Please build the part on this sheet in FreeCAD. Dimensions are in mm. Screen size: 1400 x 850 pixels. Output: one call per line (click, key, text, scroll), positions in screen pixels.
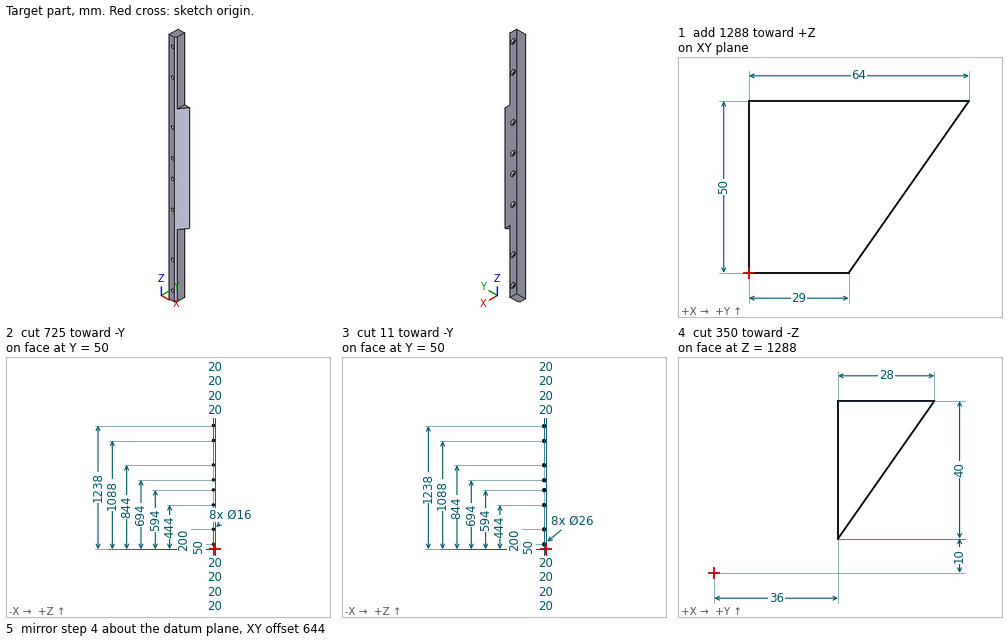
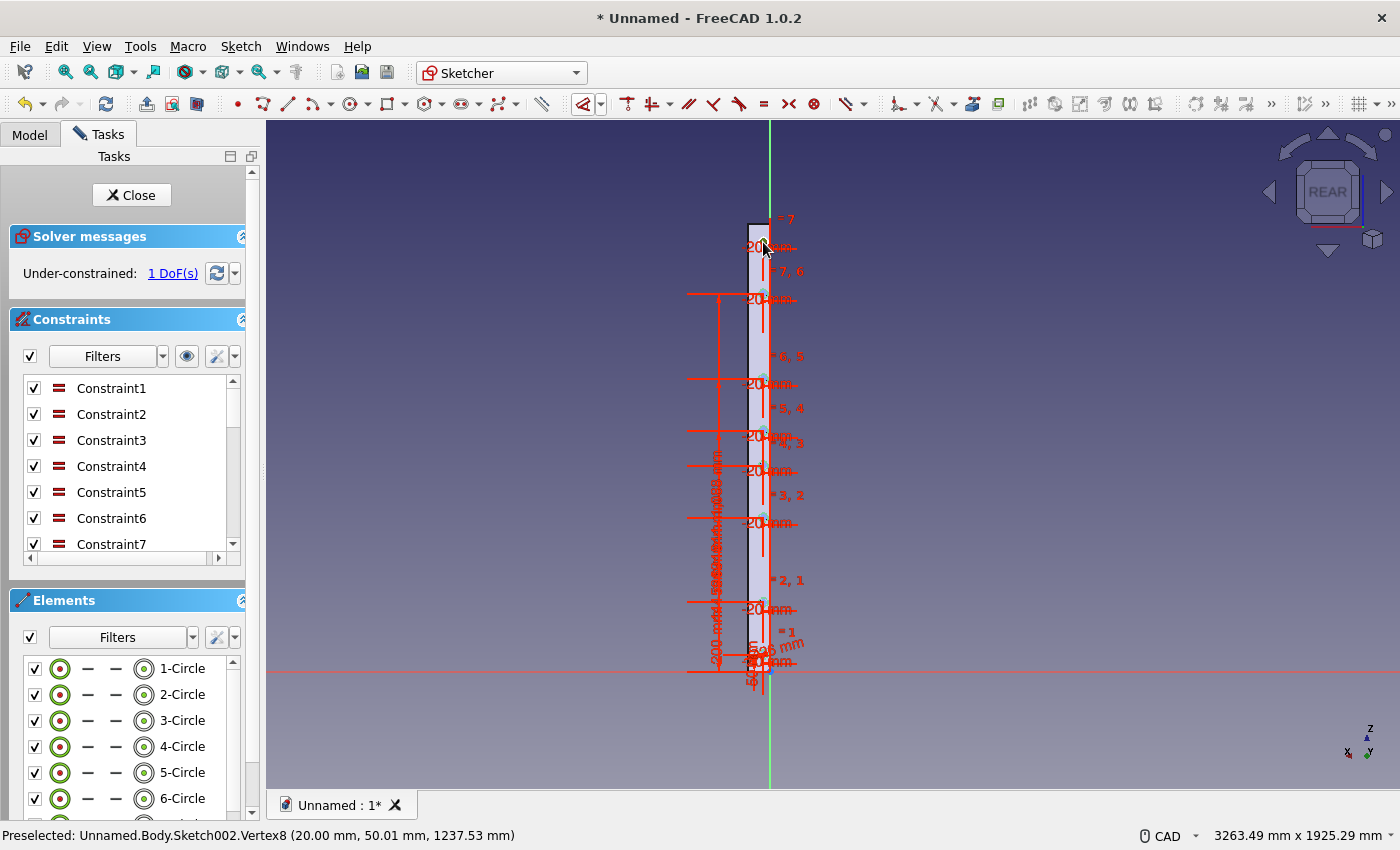
key(i)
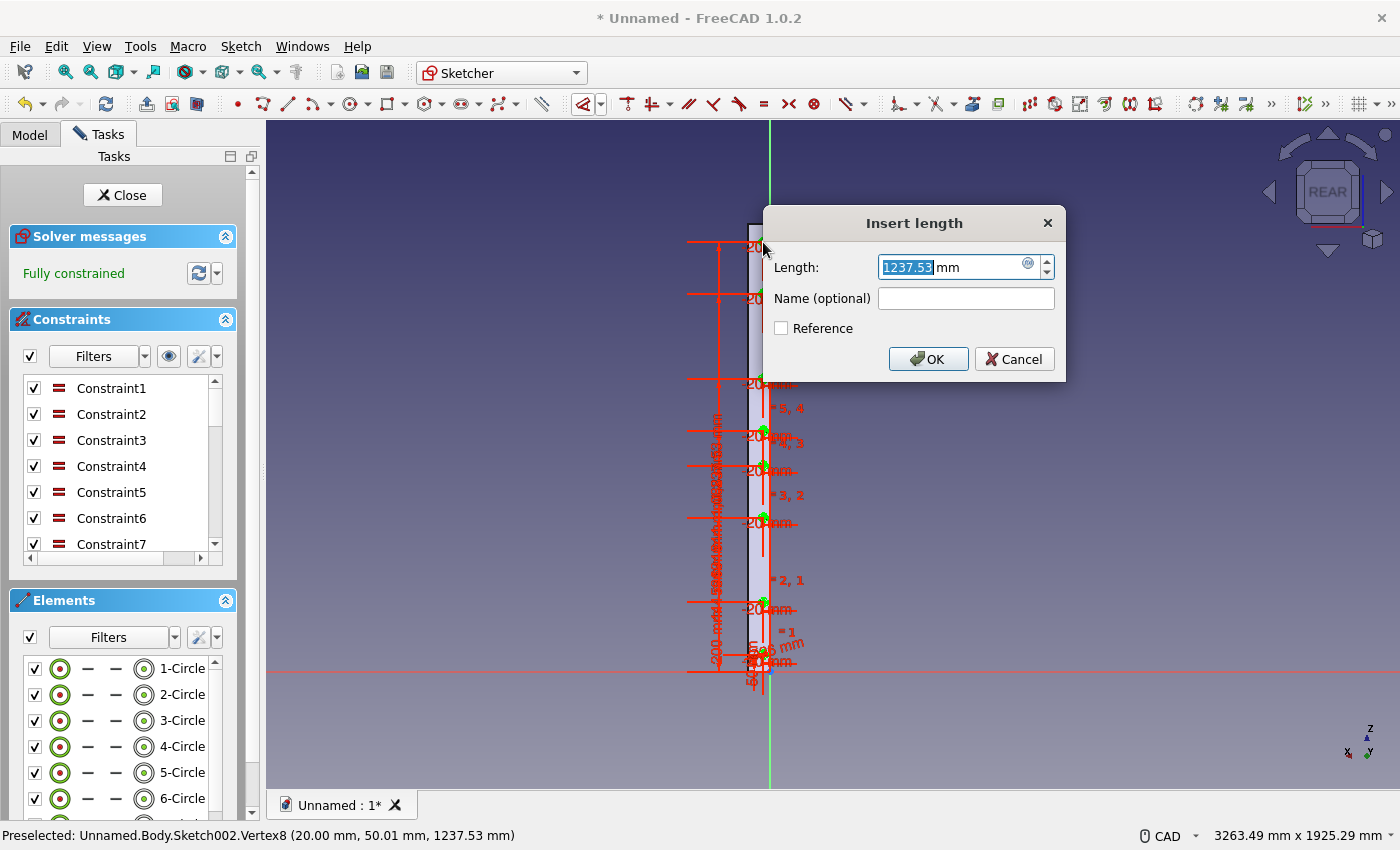
text(1238)
key(Return)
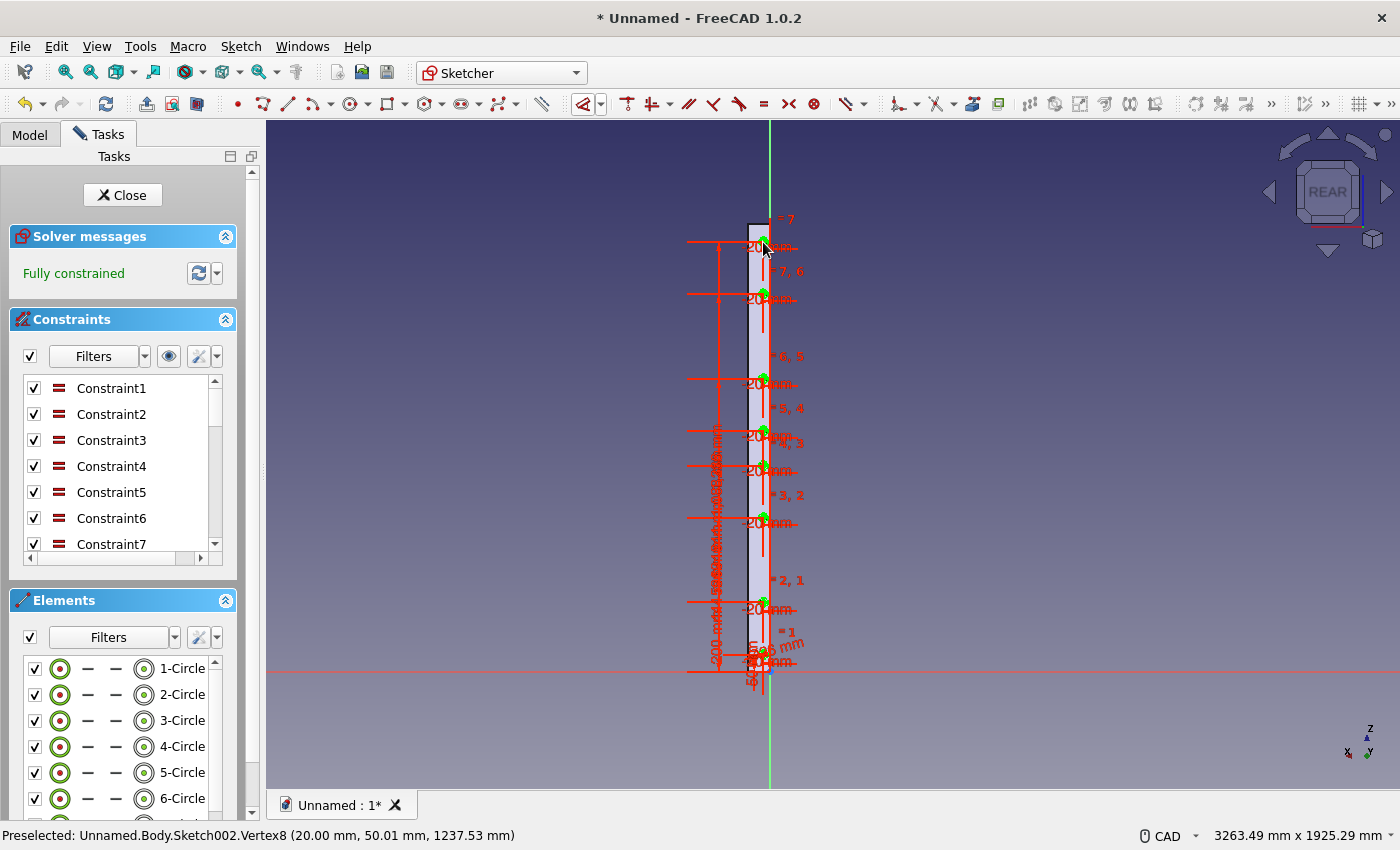
click(123, 195)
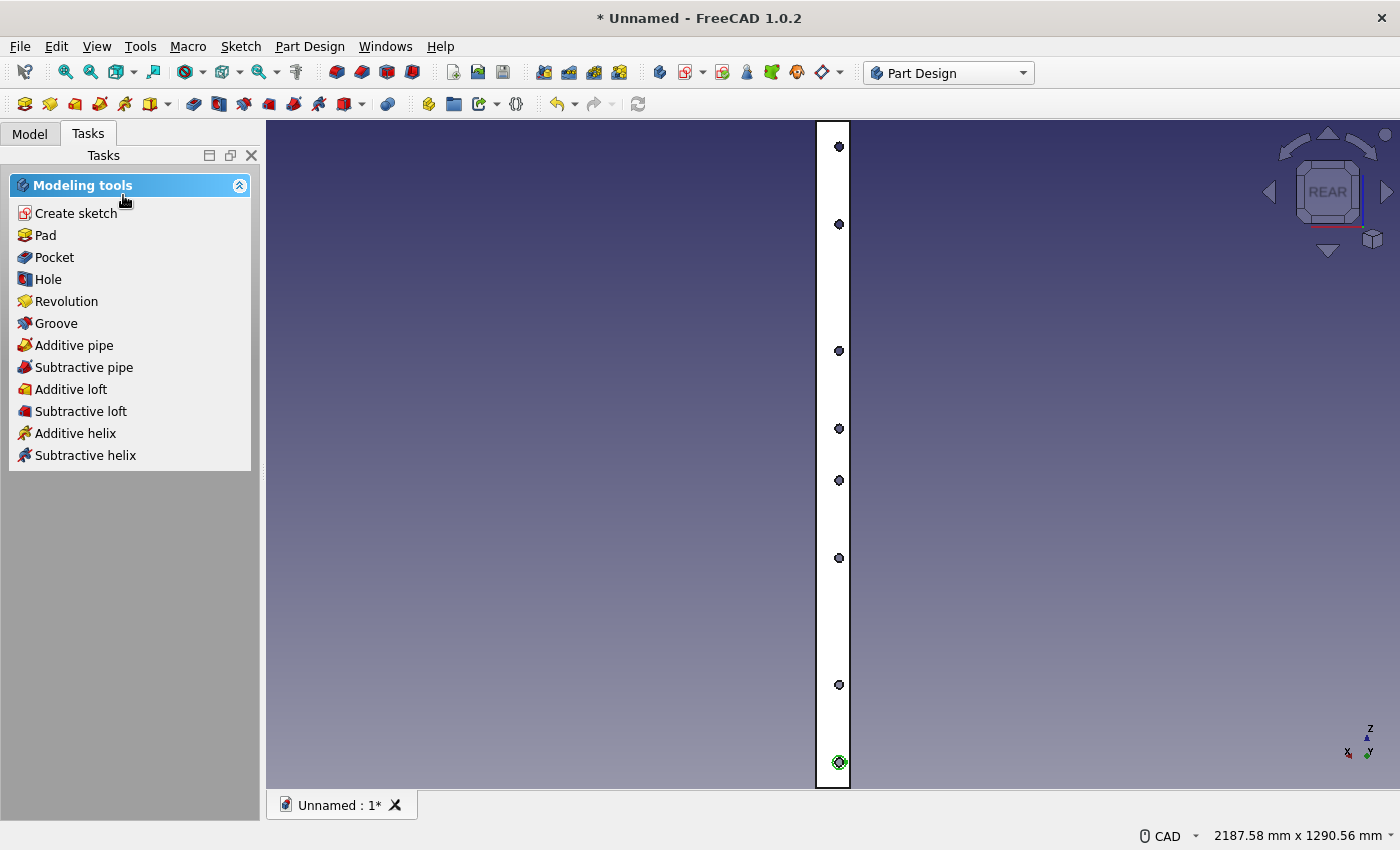
click(194, 104)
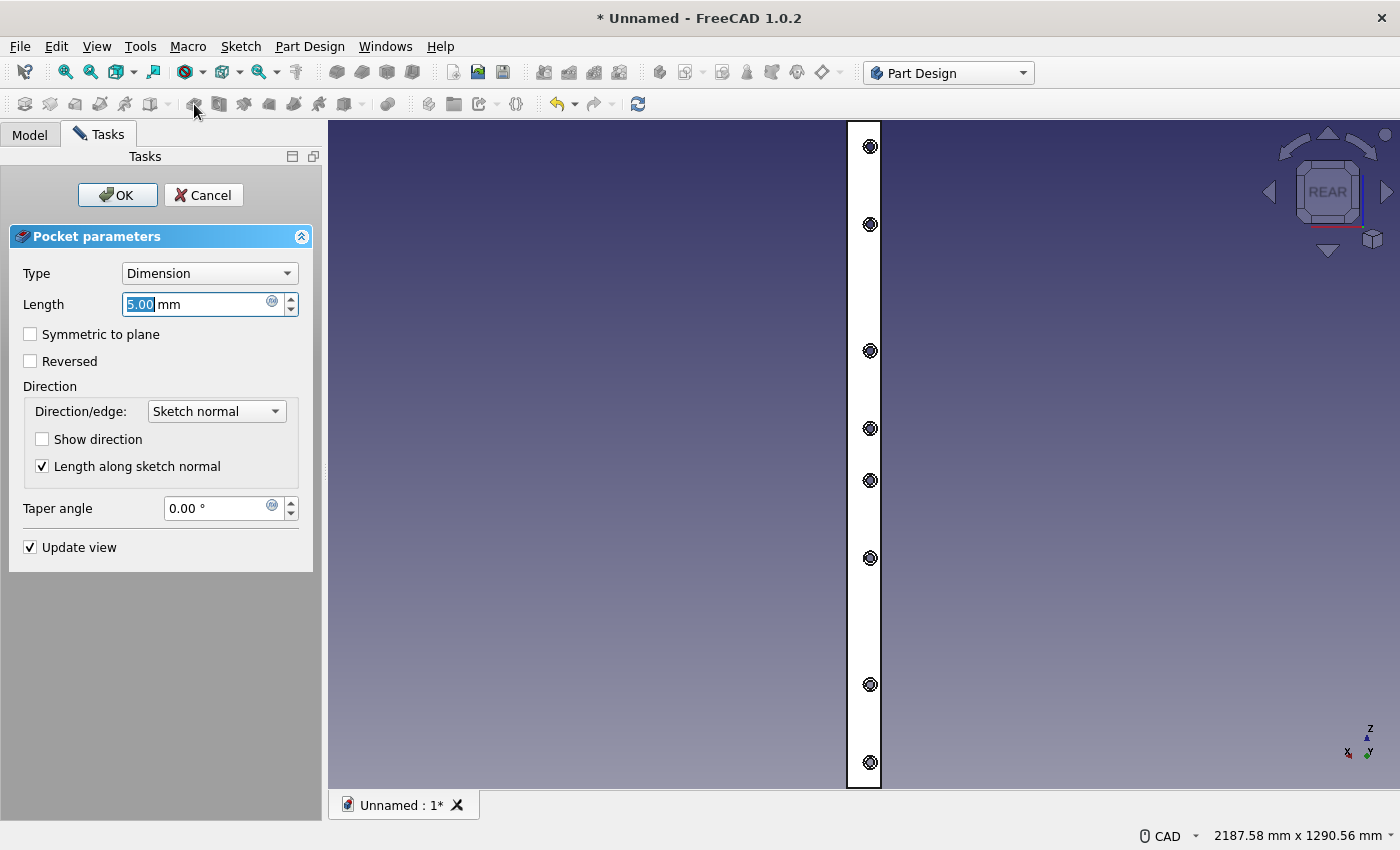
text(11)
key(Tab)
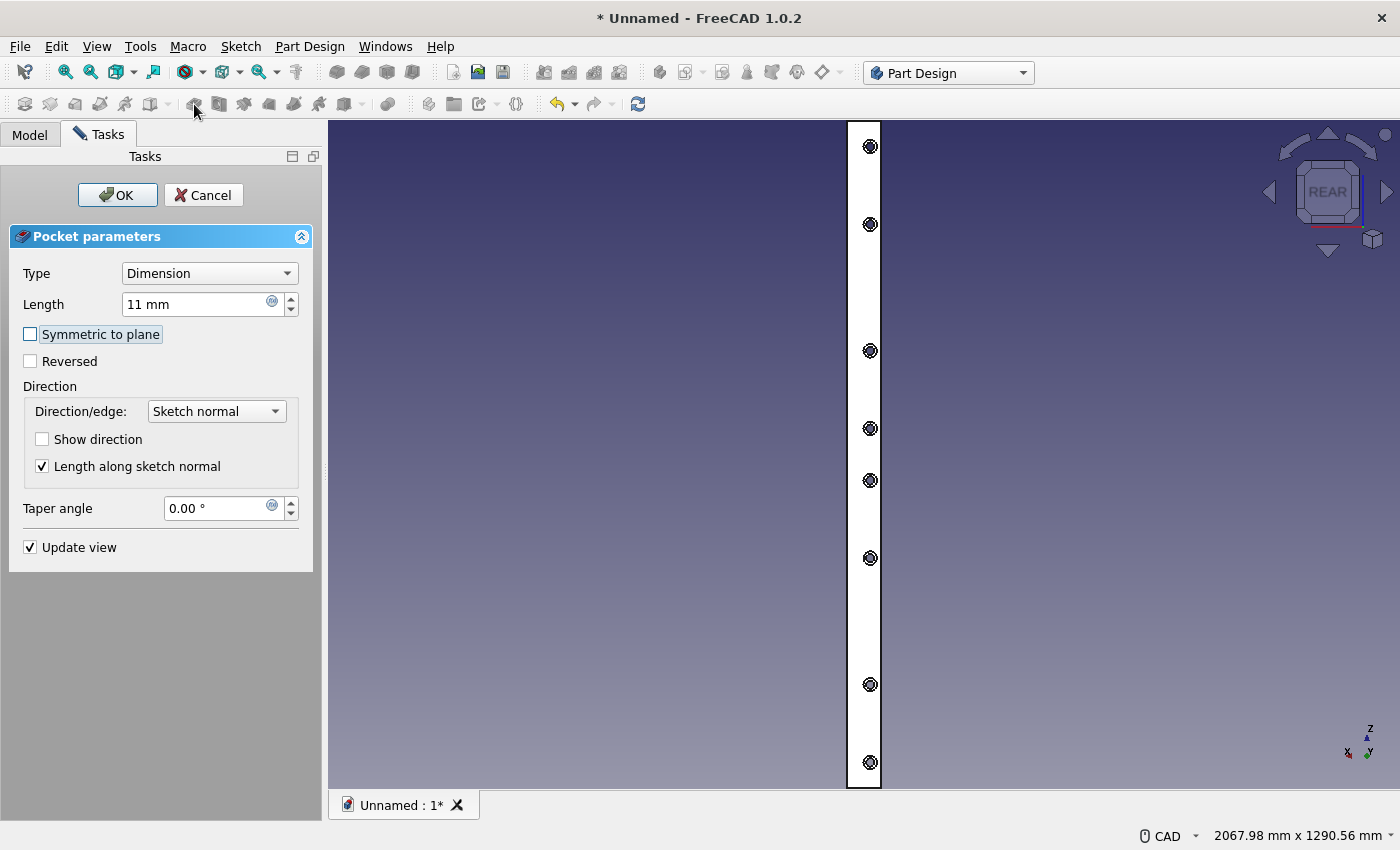
click(118, 195)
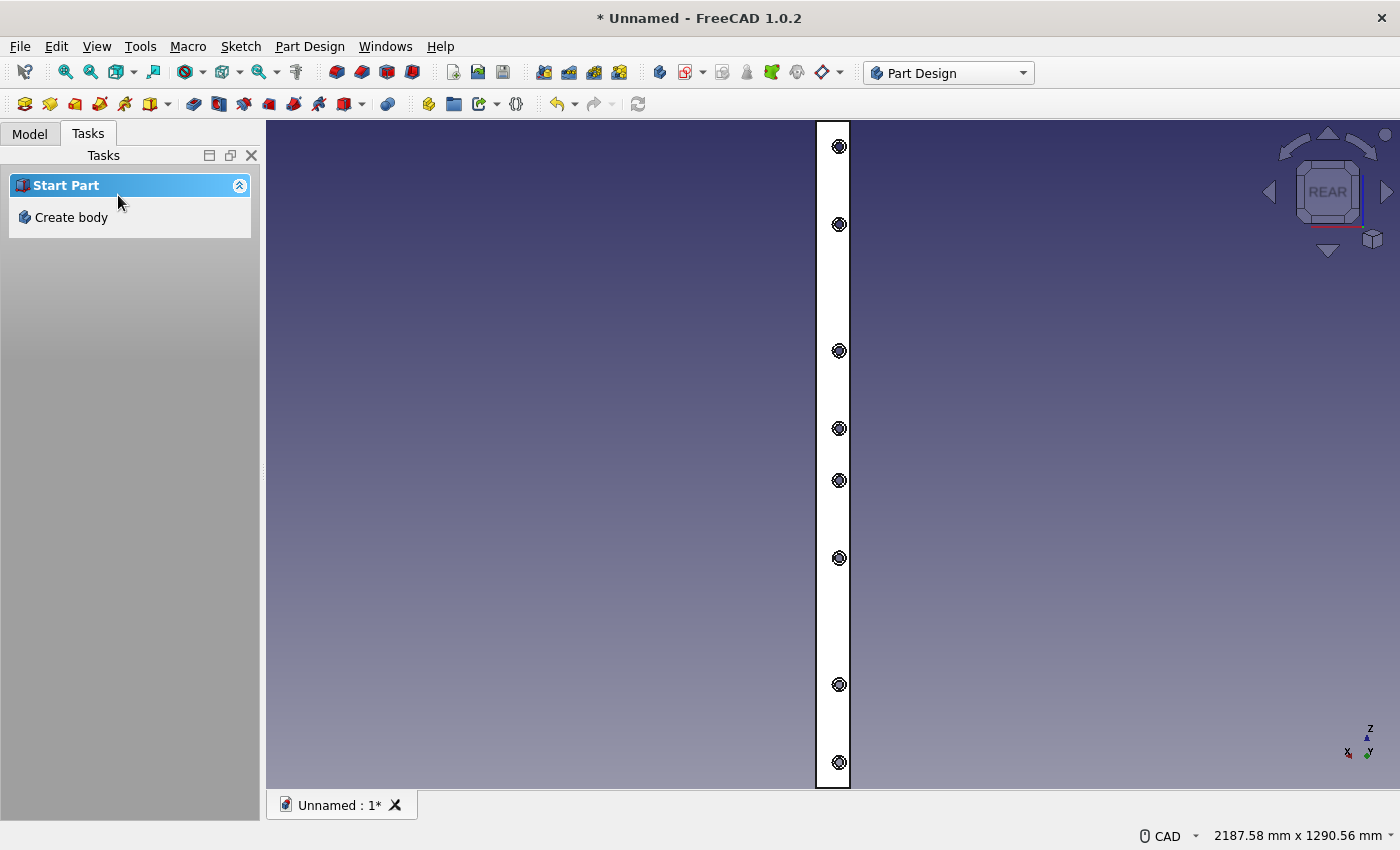
key(0)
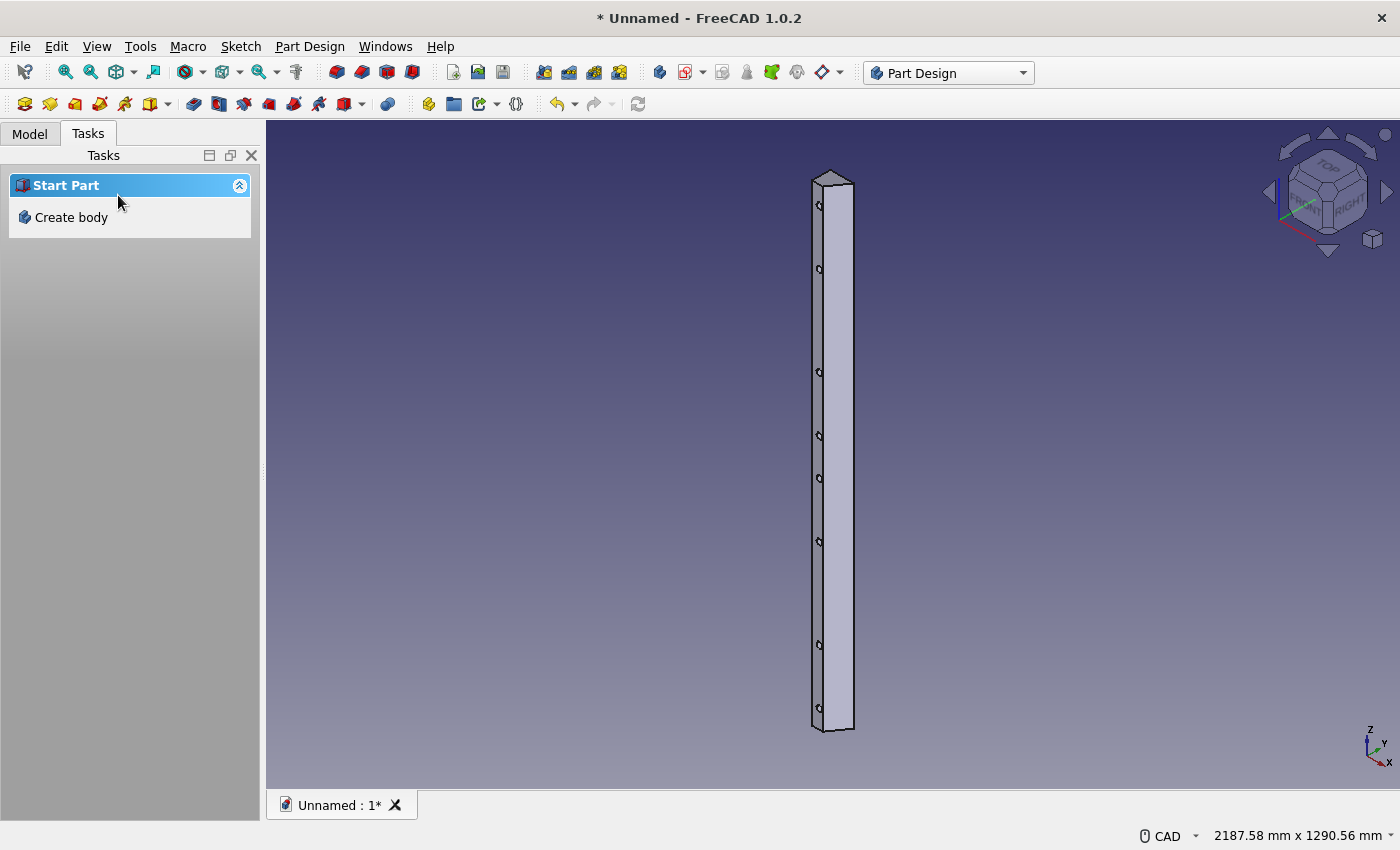
click(829, 176)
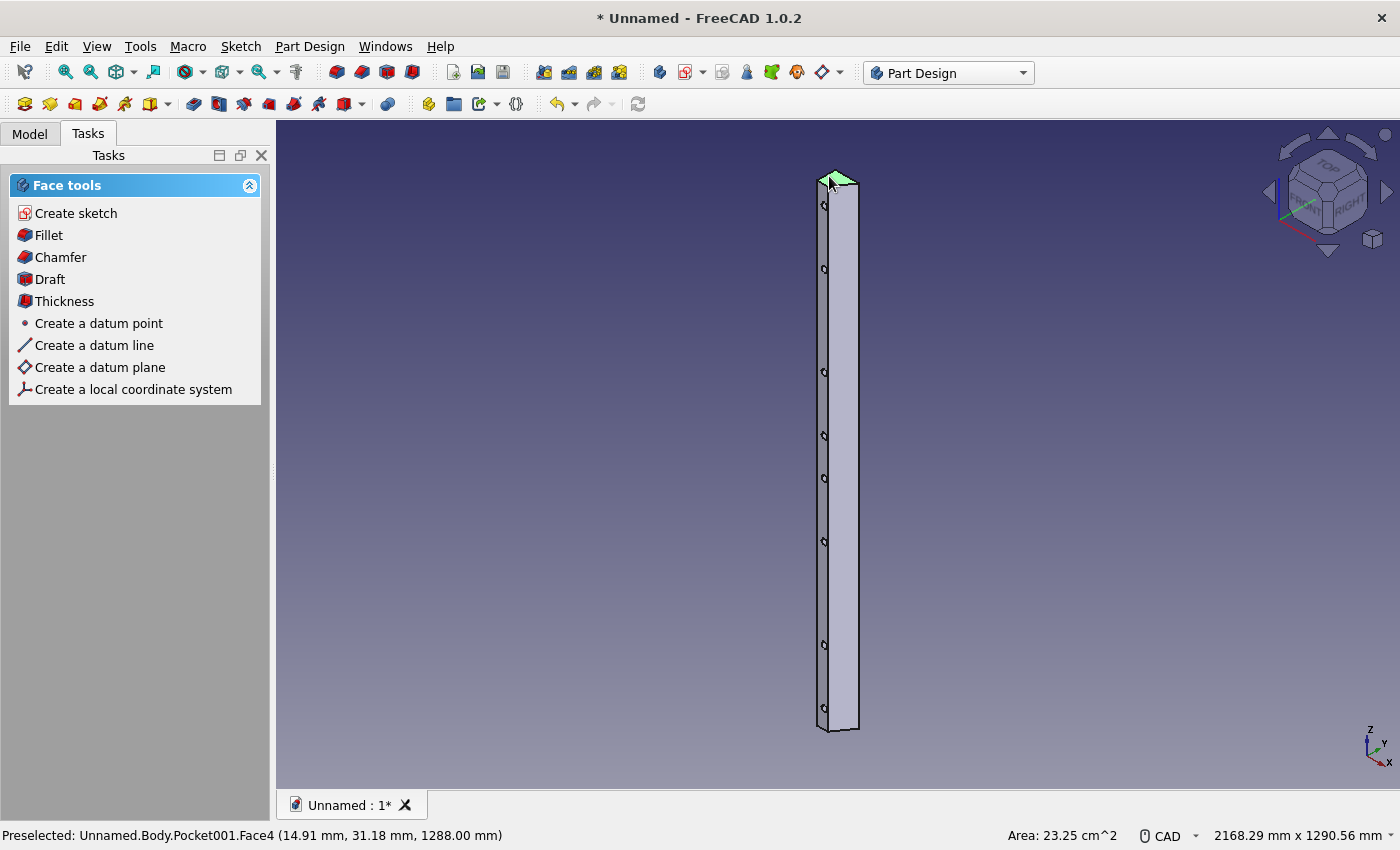
click(684, 72)